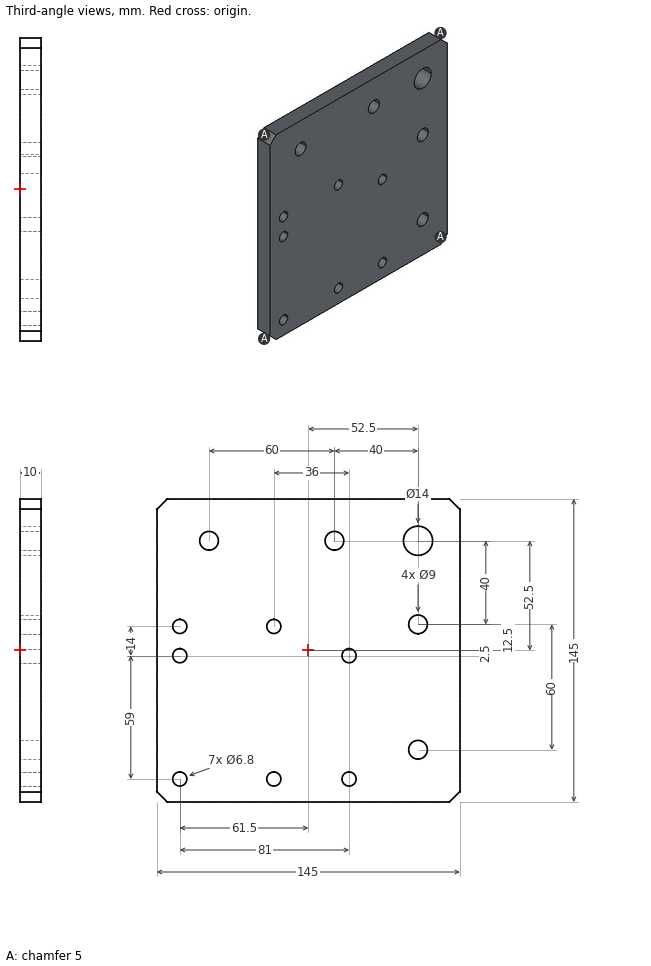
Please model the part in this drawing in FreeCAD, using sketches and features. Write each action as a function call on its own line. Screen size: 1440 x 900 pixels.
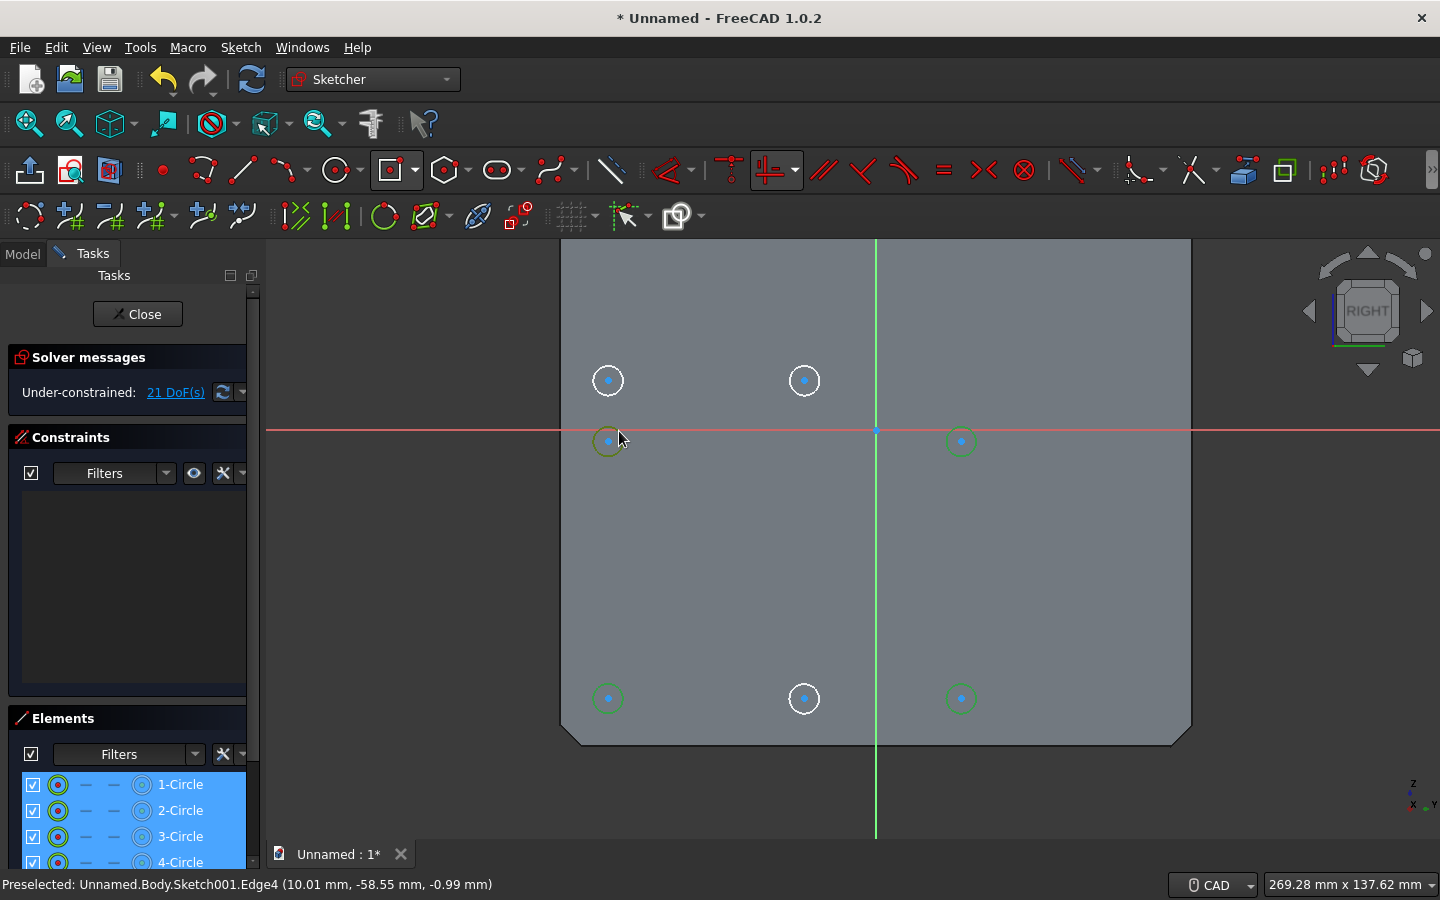
click(619, 370)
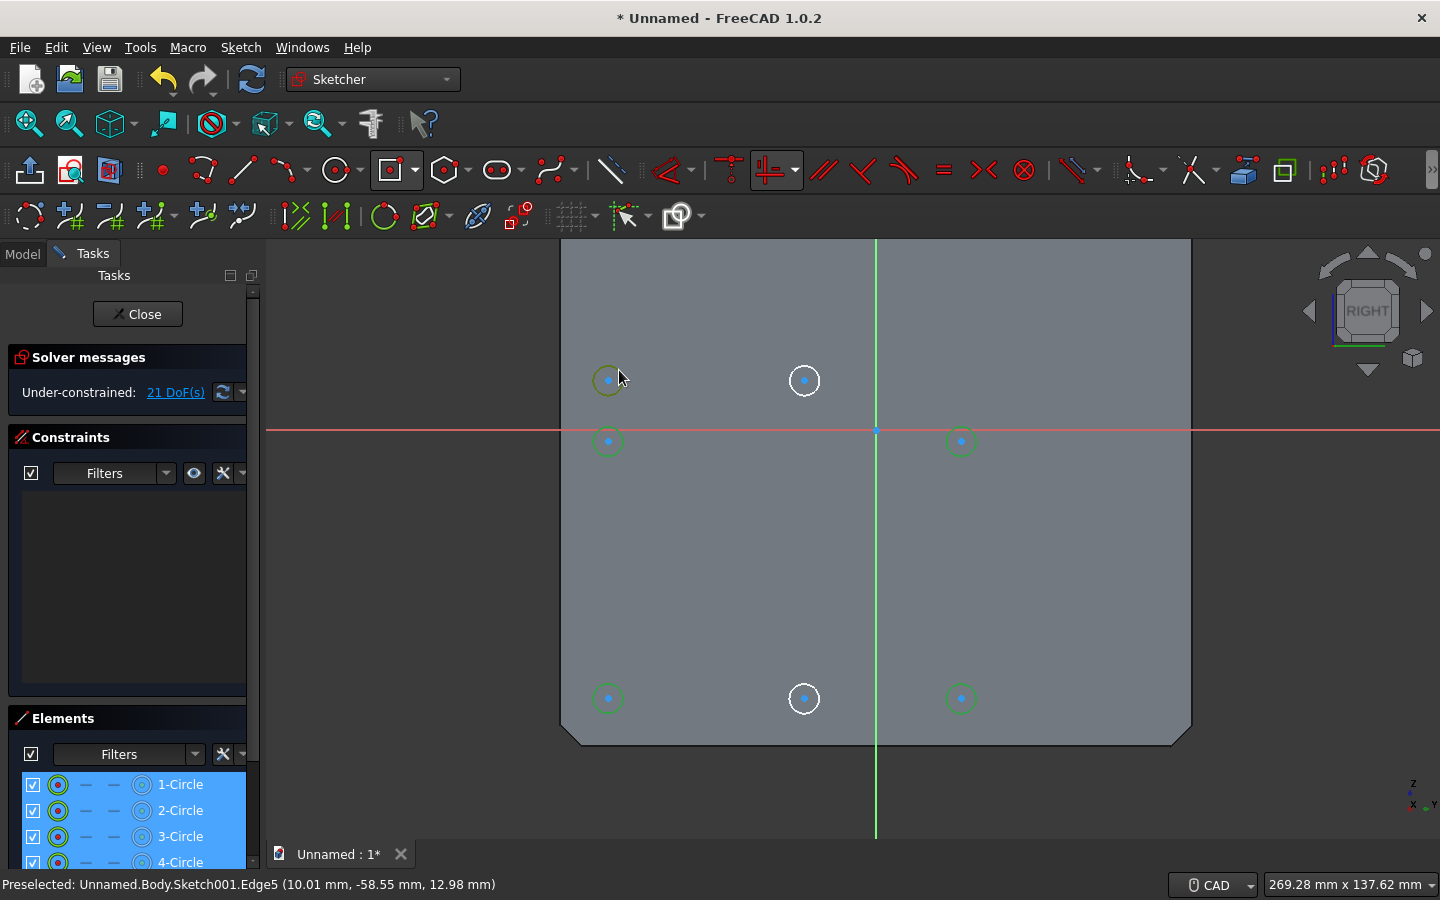
click(815, 370)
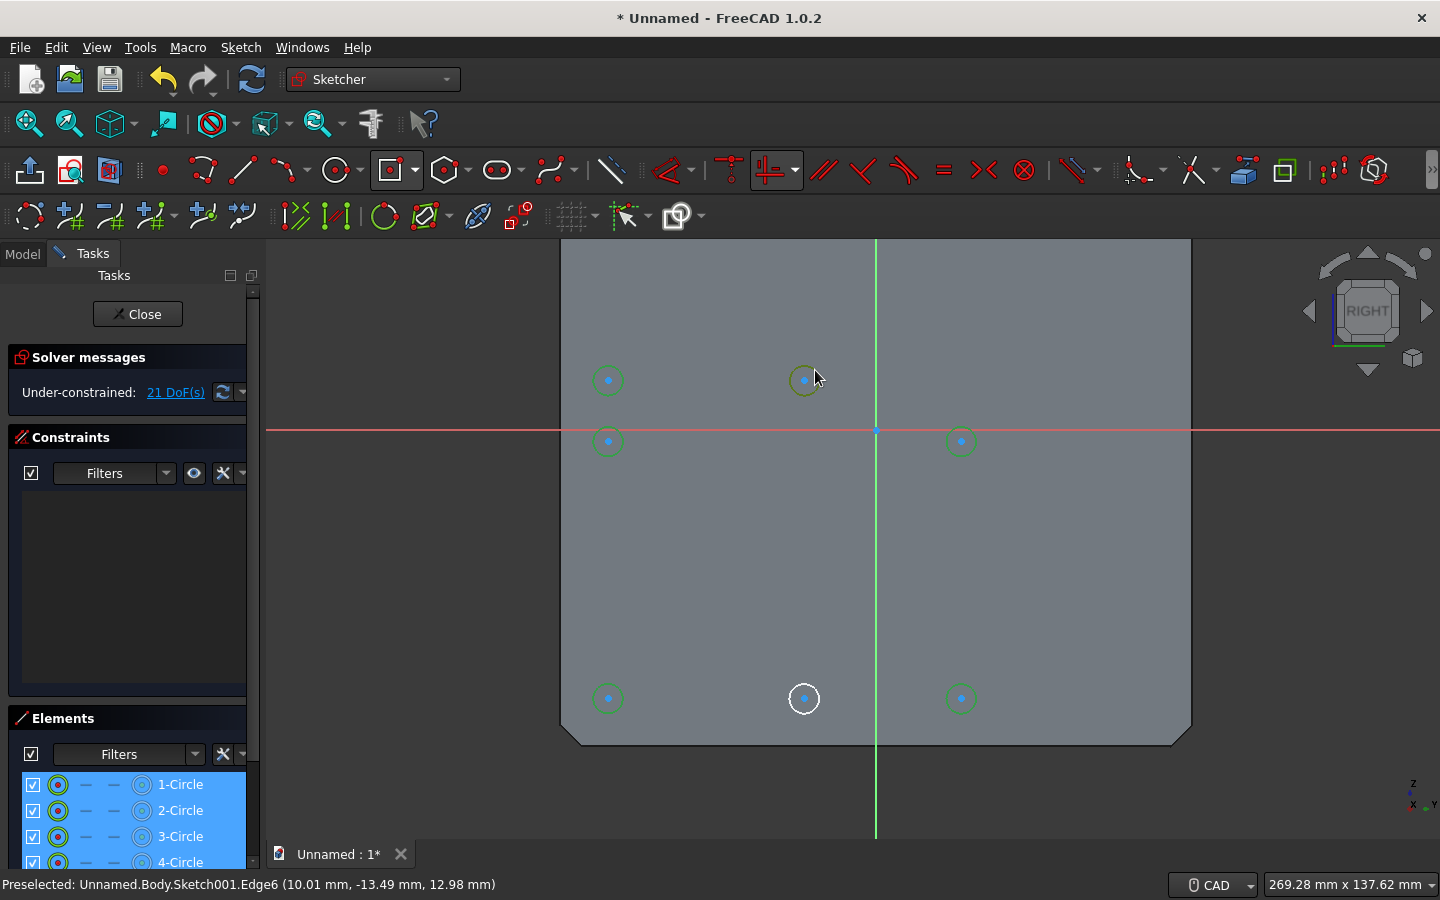
click(815, 688)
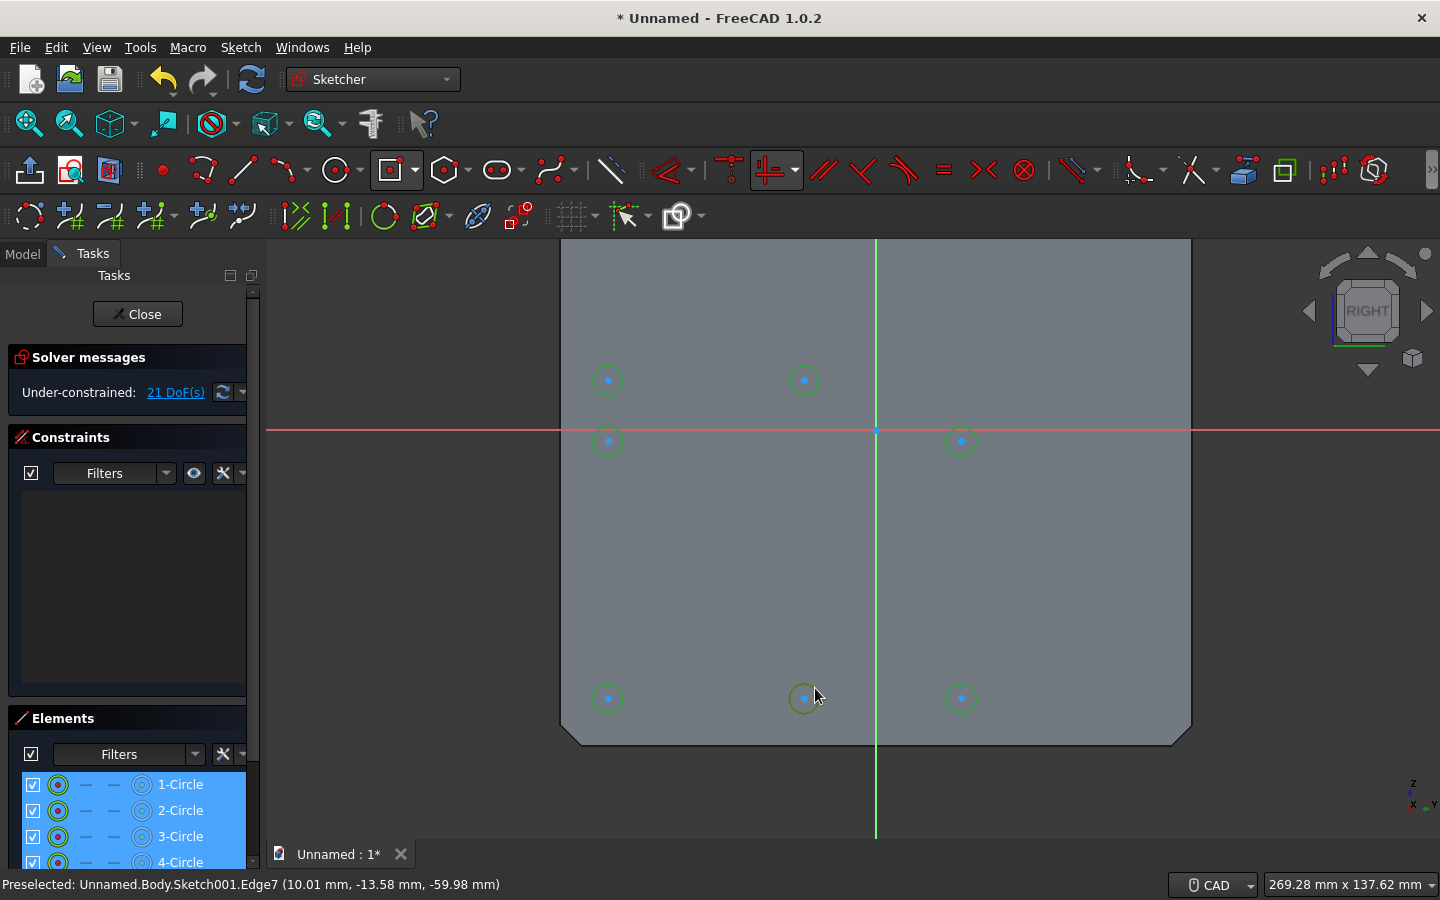
key(e)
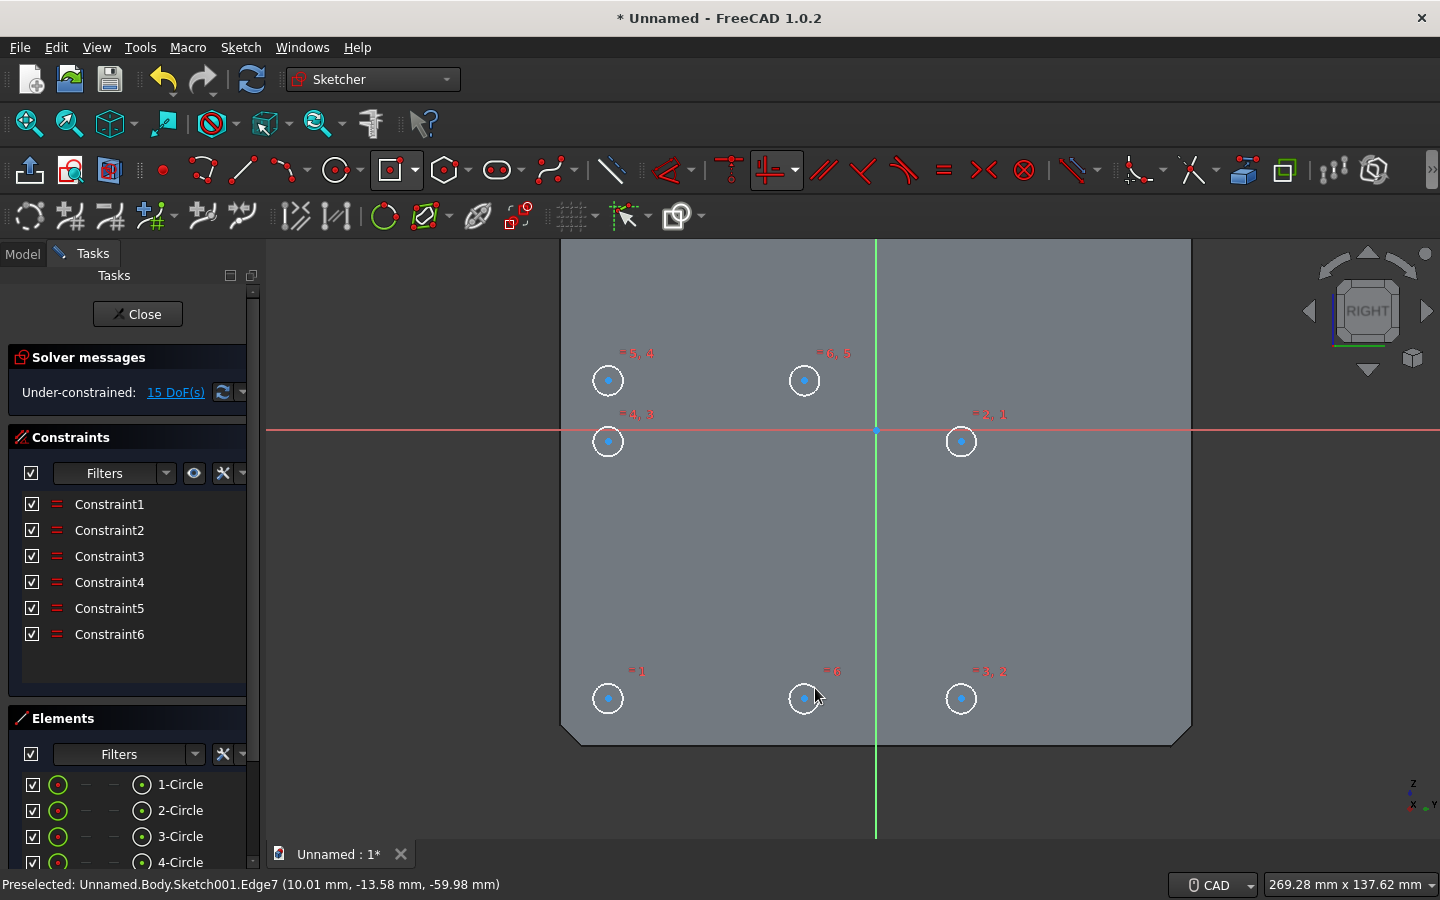
click(961, 442)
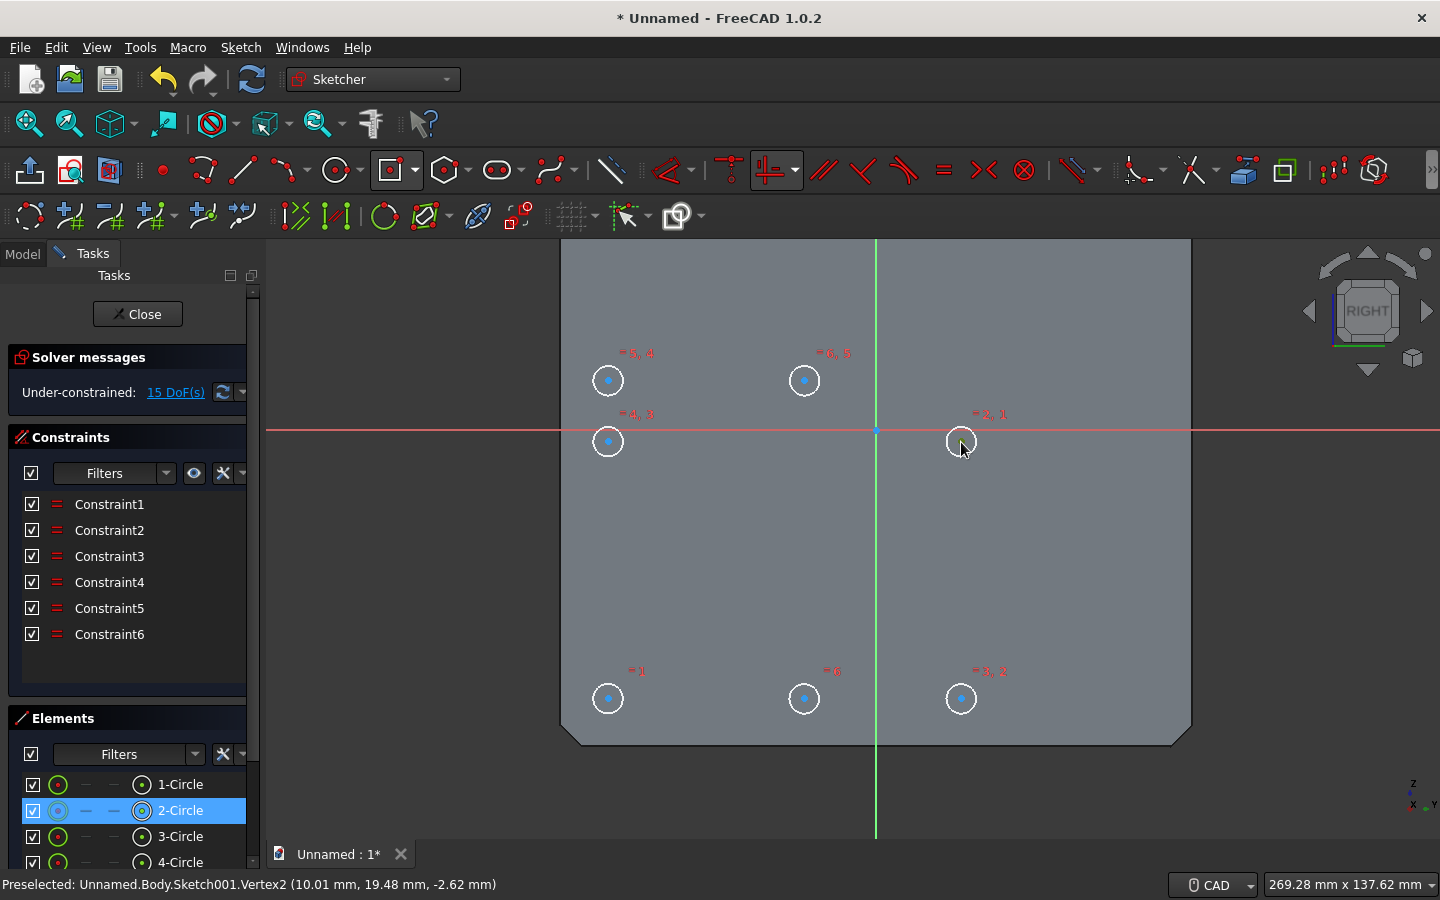
click(961, 699)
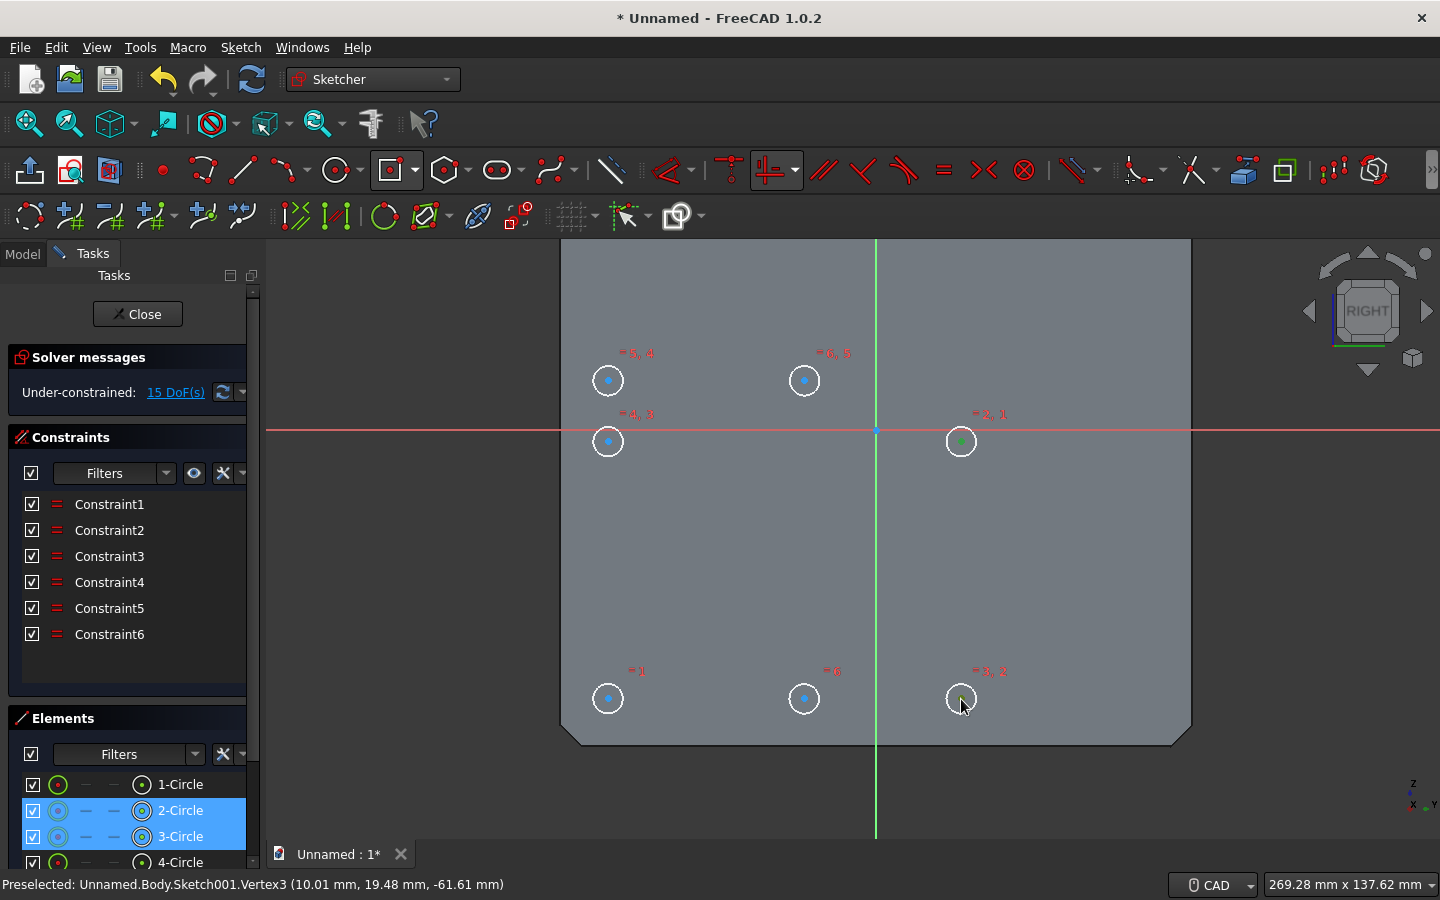
click(798, 170)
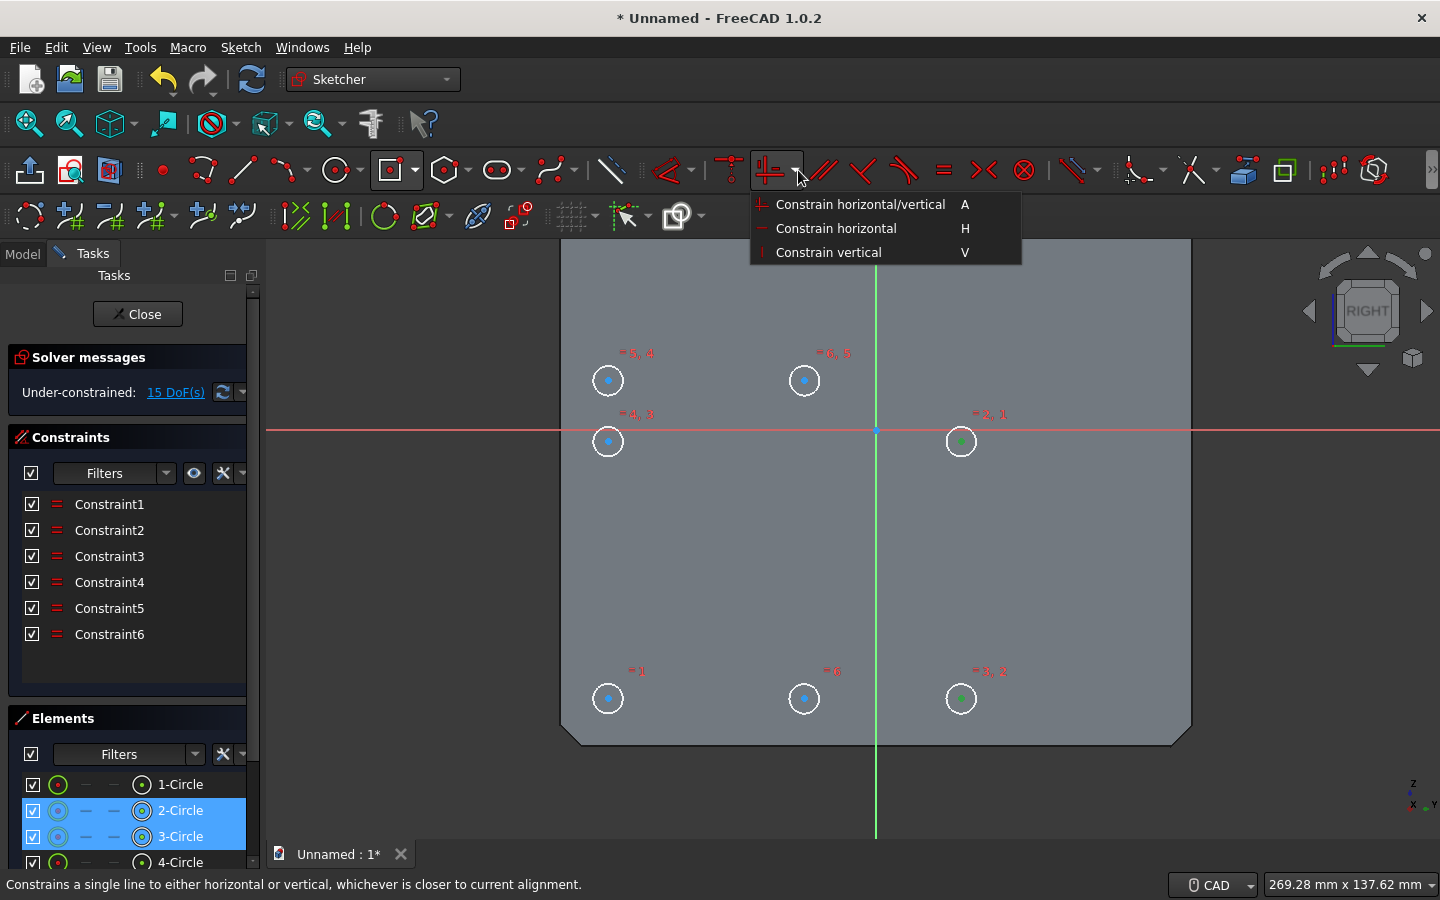
click(886, 252)